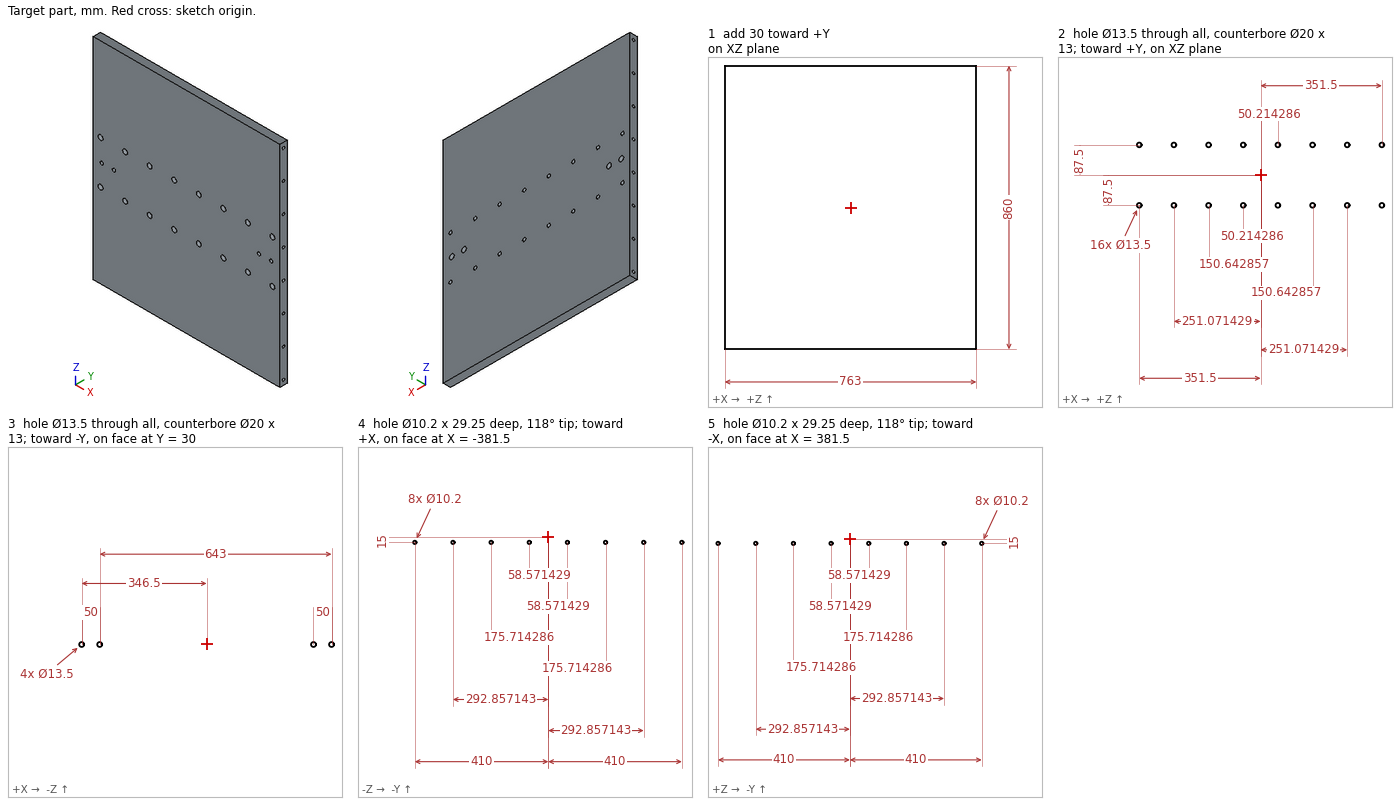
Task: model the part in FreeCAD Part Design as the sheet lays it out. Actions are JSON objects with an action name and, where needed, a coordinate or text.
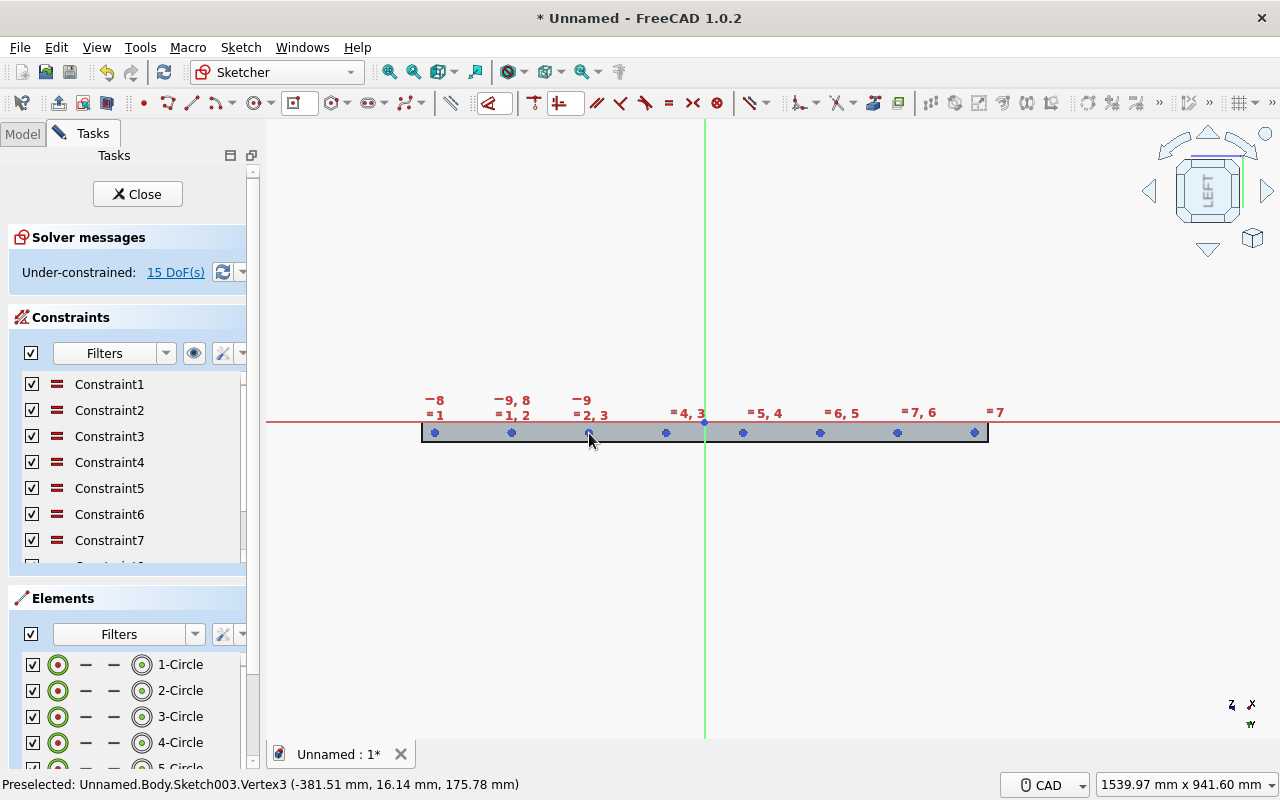
{"action": "left_click", "coordinate": [589, 433]}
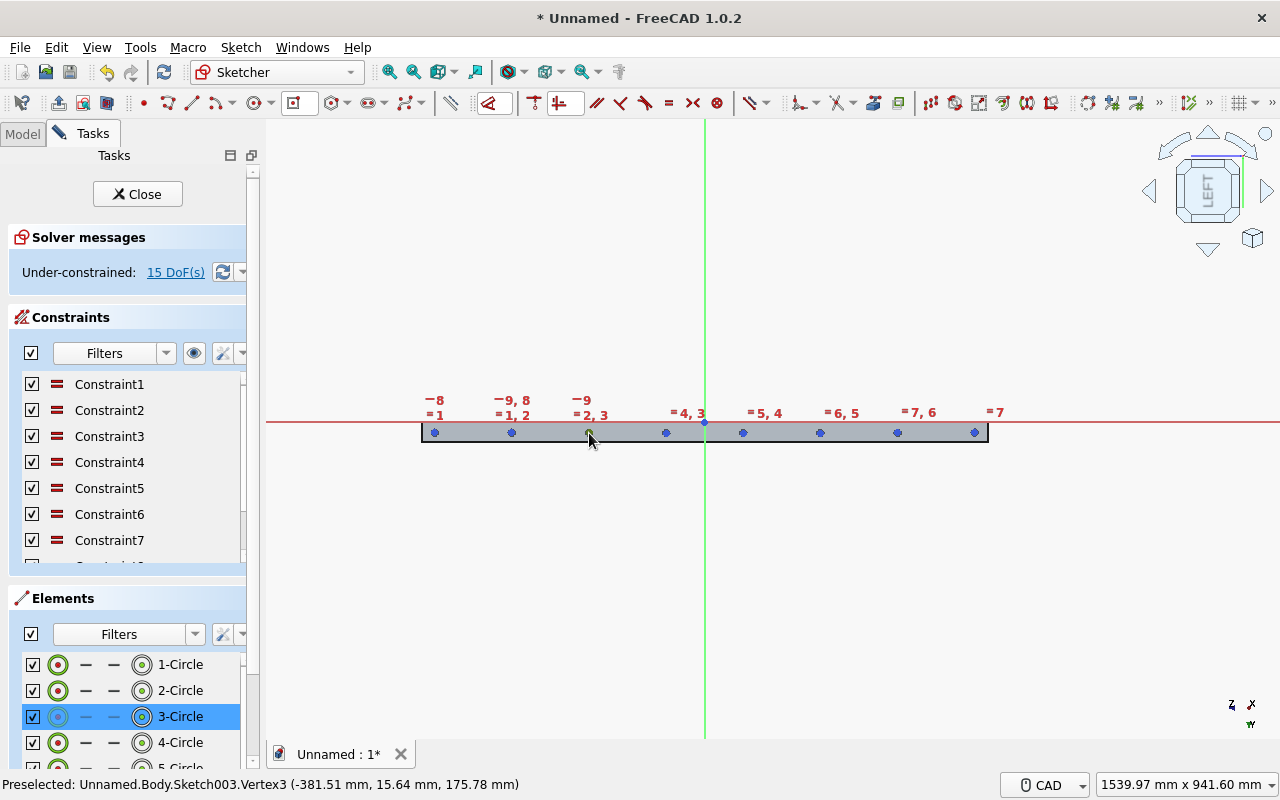
{"action": "left_click", "coordinate": [666, 433]}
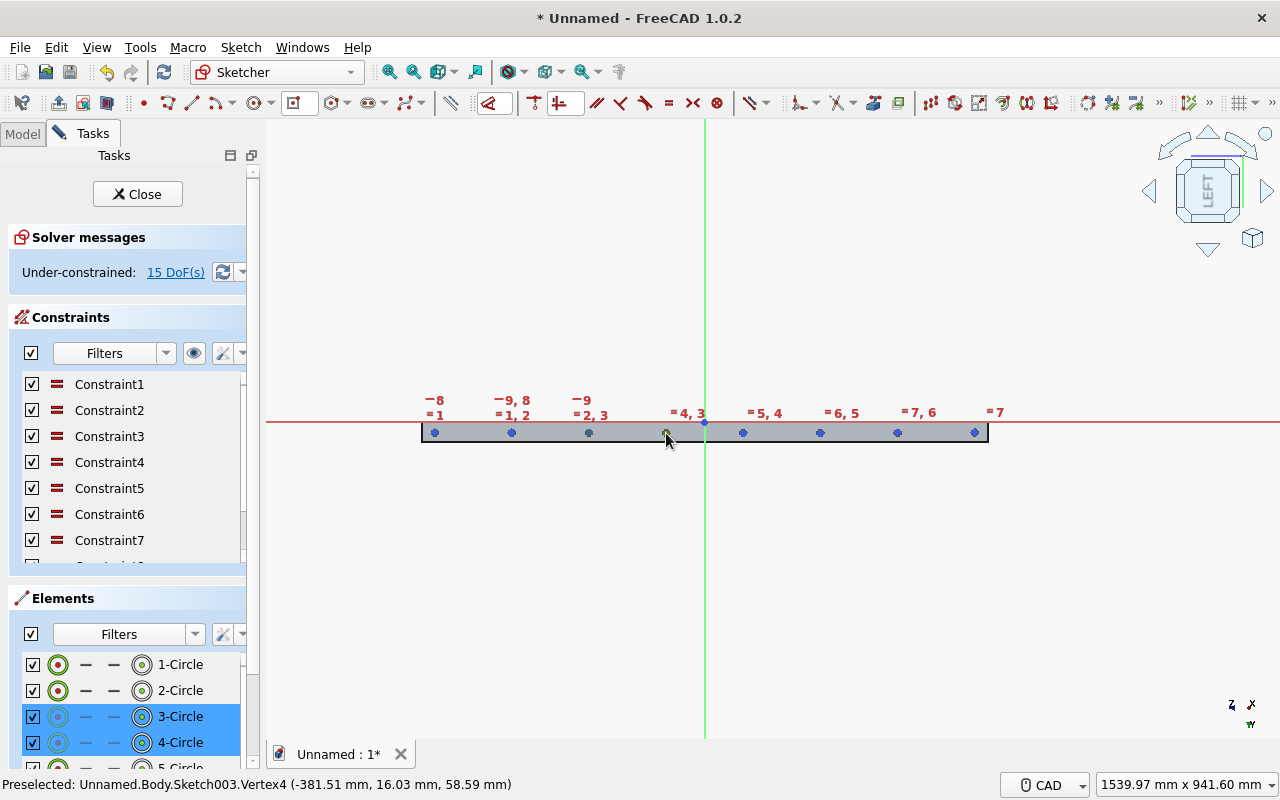
{"action": "left_click", "coordinate": [578, 104]}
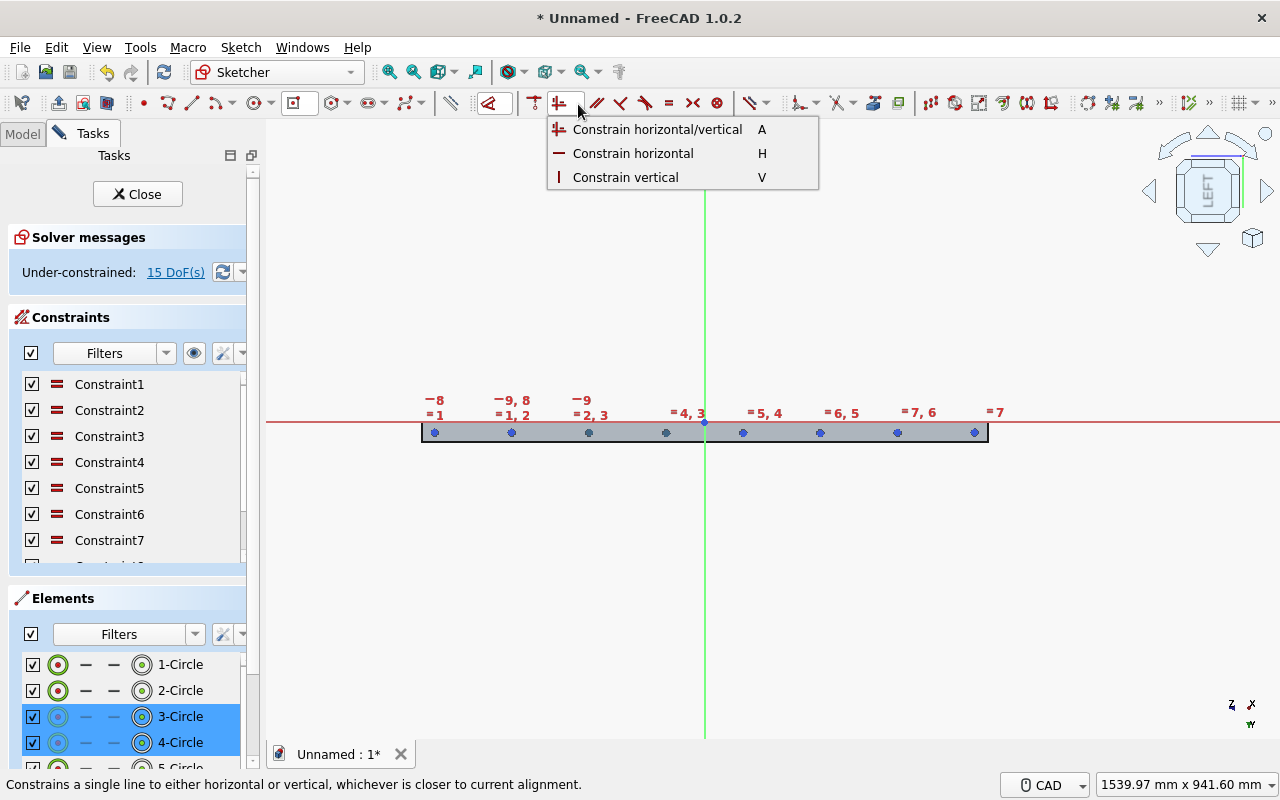
{"action": "left_click", "coordinate": [683, 153]}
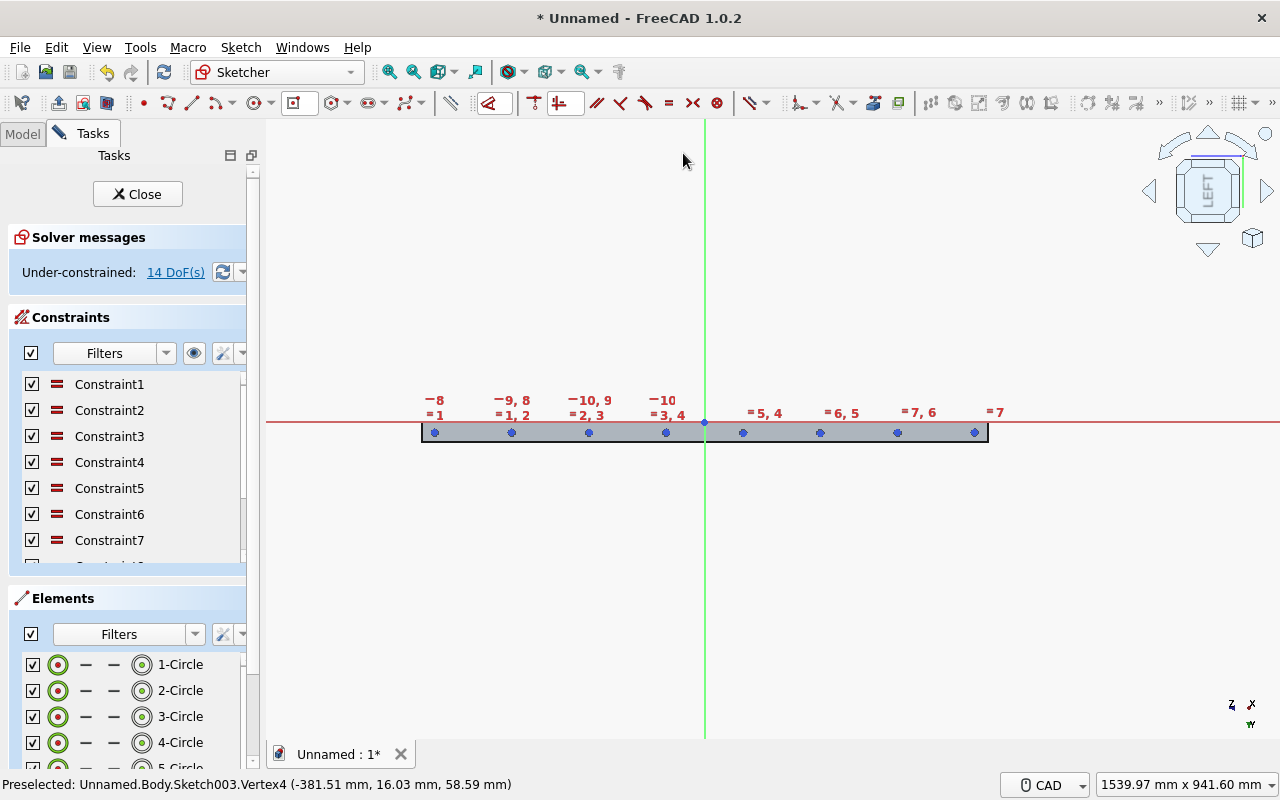
{"action": "left_click", "coordinate": [666, 433]}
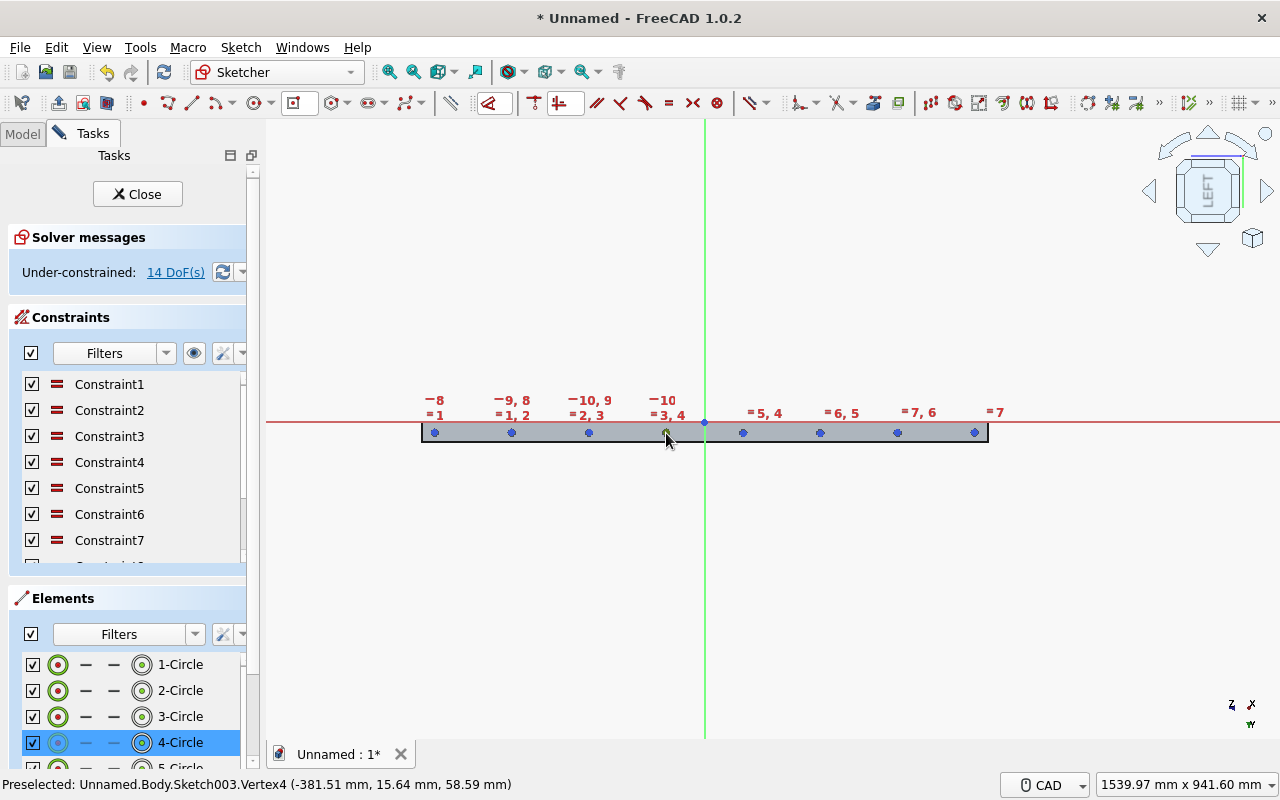
{"action": "left_click", "coordinate": [743, 433]}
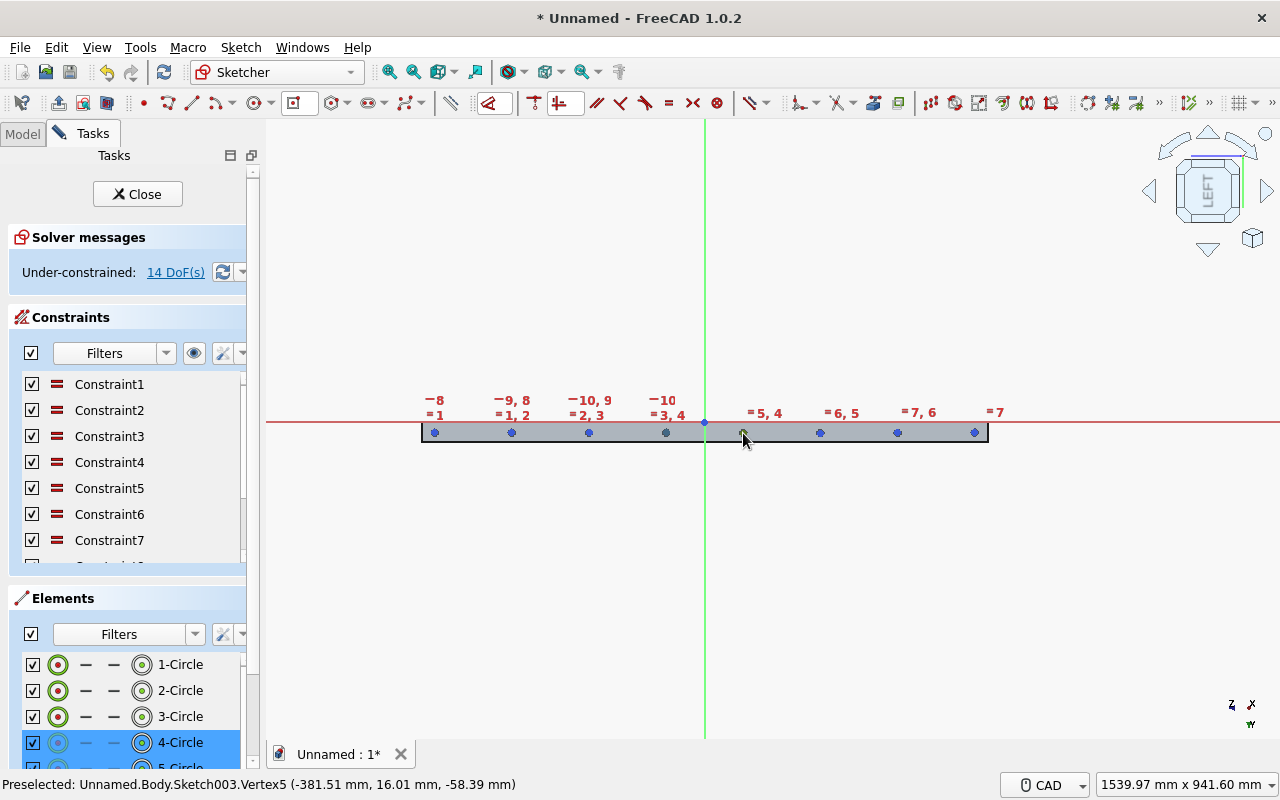
{"action": "left_click", "coordinate": [578, 104]}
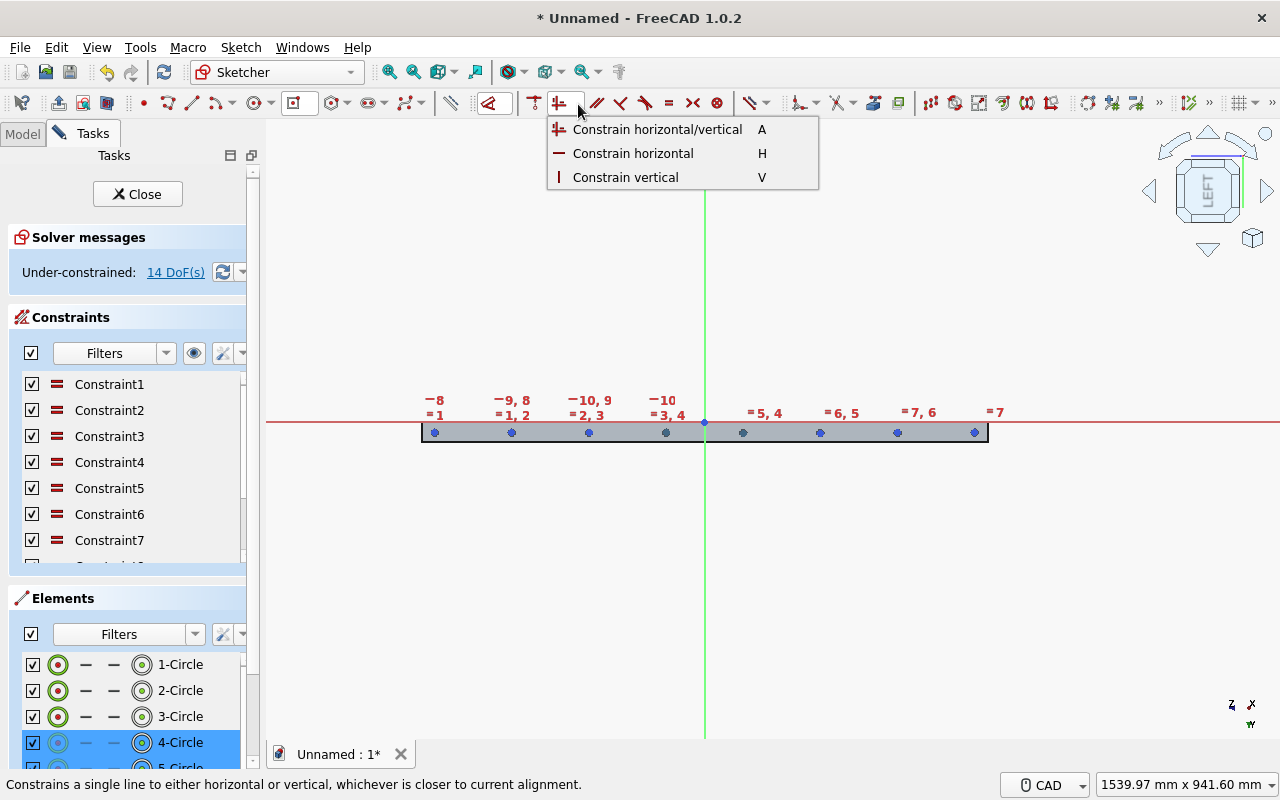
{"action": "left_click", "coordinate": [683, 153]}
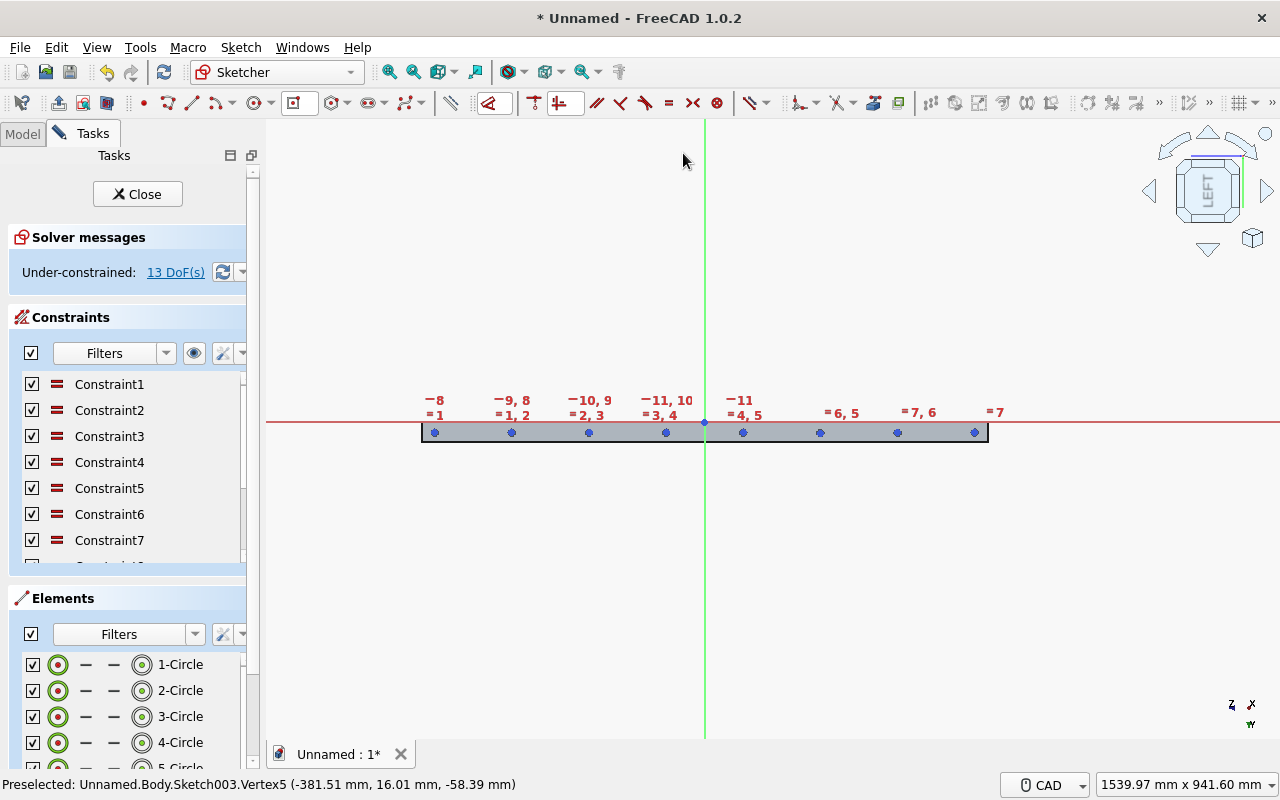
{"action": "left_click", "coordinate": [743, 433]}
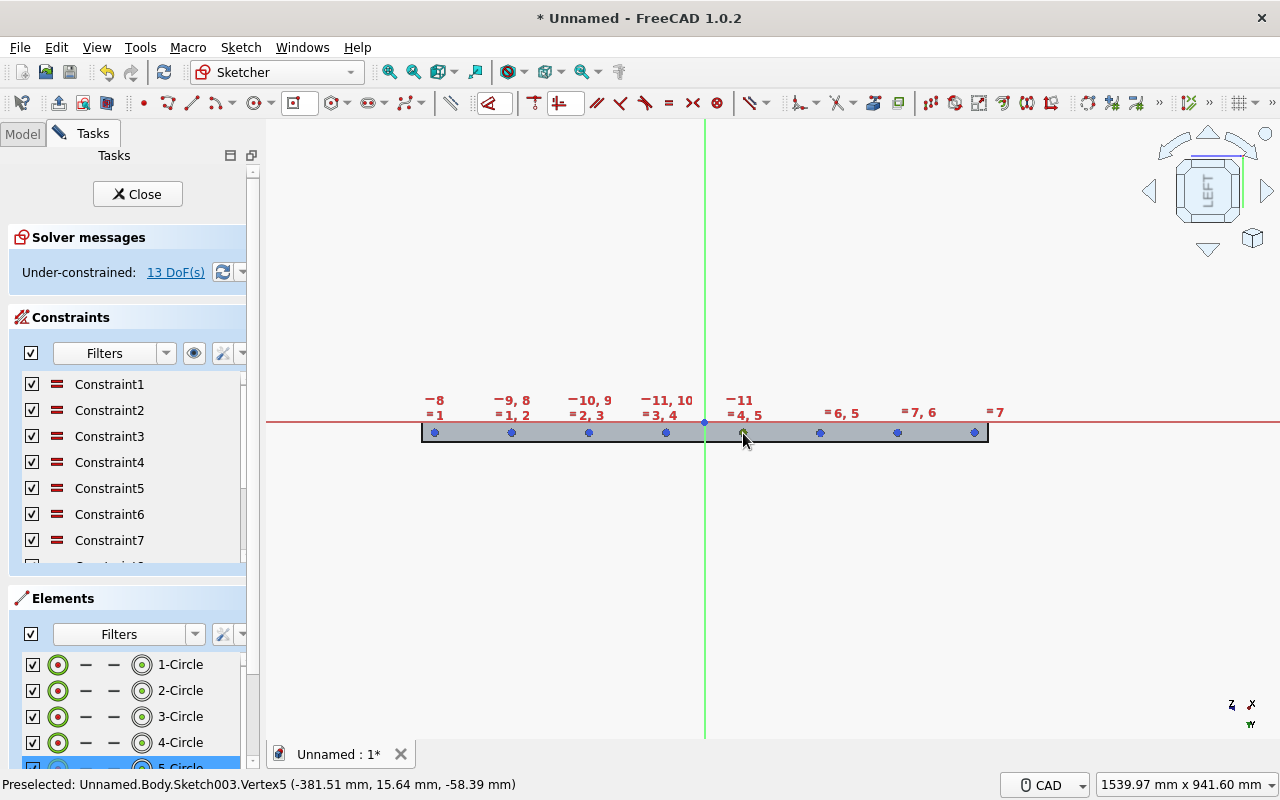
{"action": "left_click", "coordinate": [820, 433]}